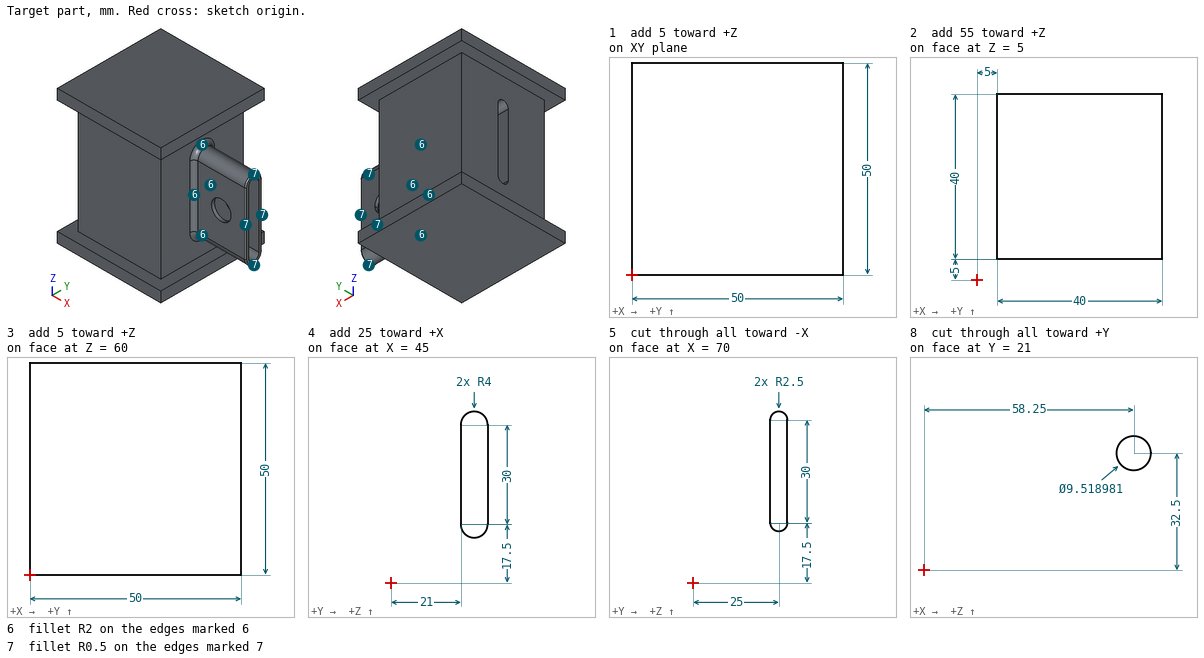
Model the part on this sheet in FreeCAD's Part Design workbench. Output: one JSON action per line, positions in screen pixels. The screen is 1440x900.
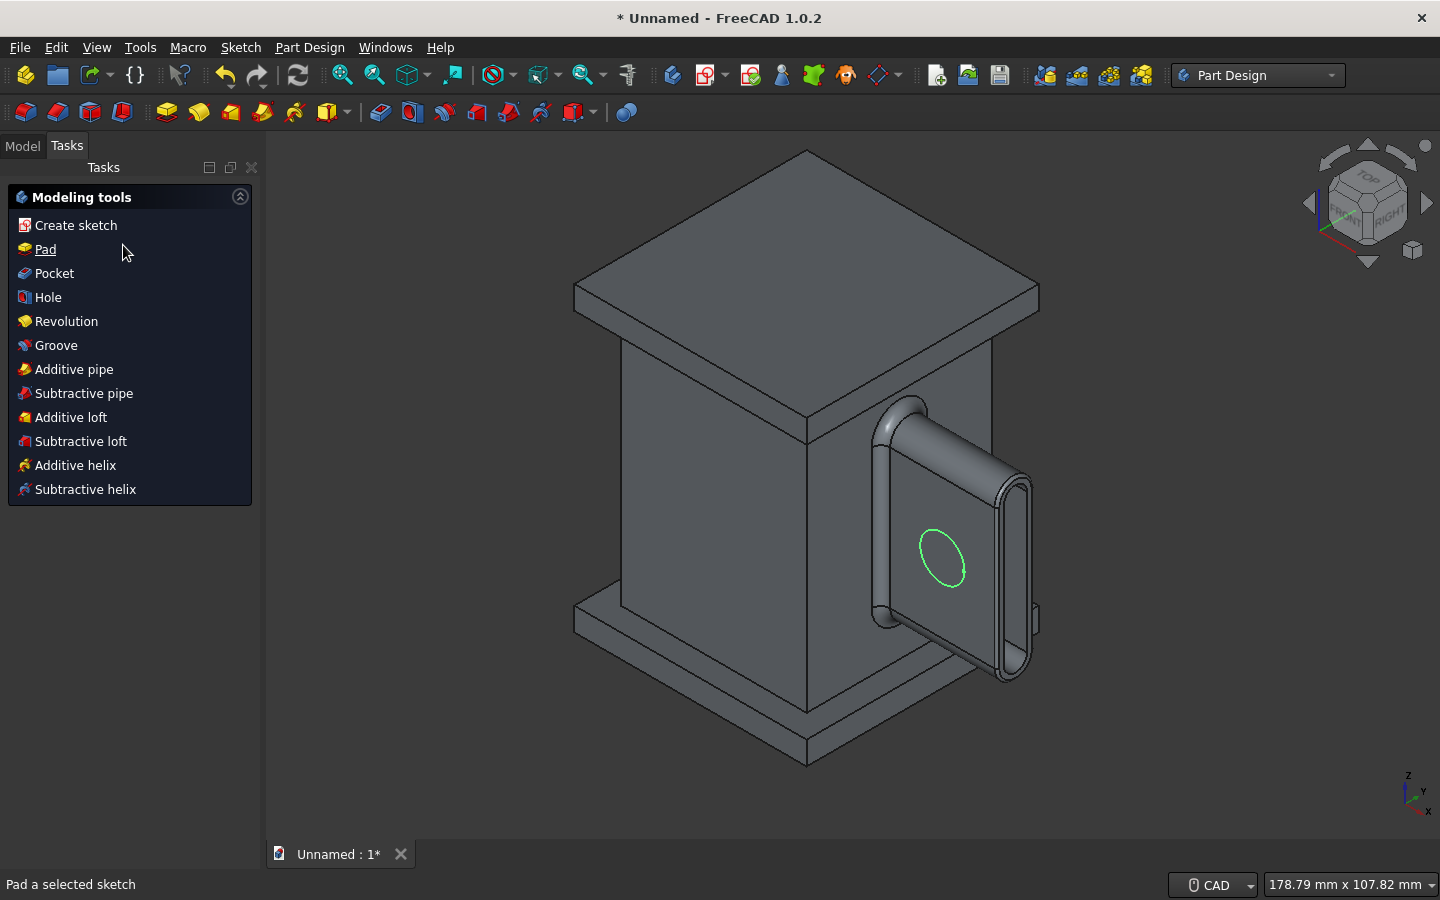
{"action": "left_click", "coordinate": [382, 112]}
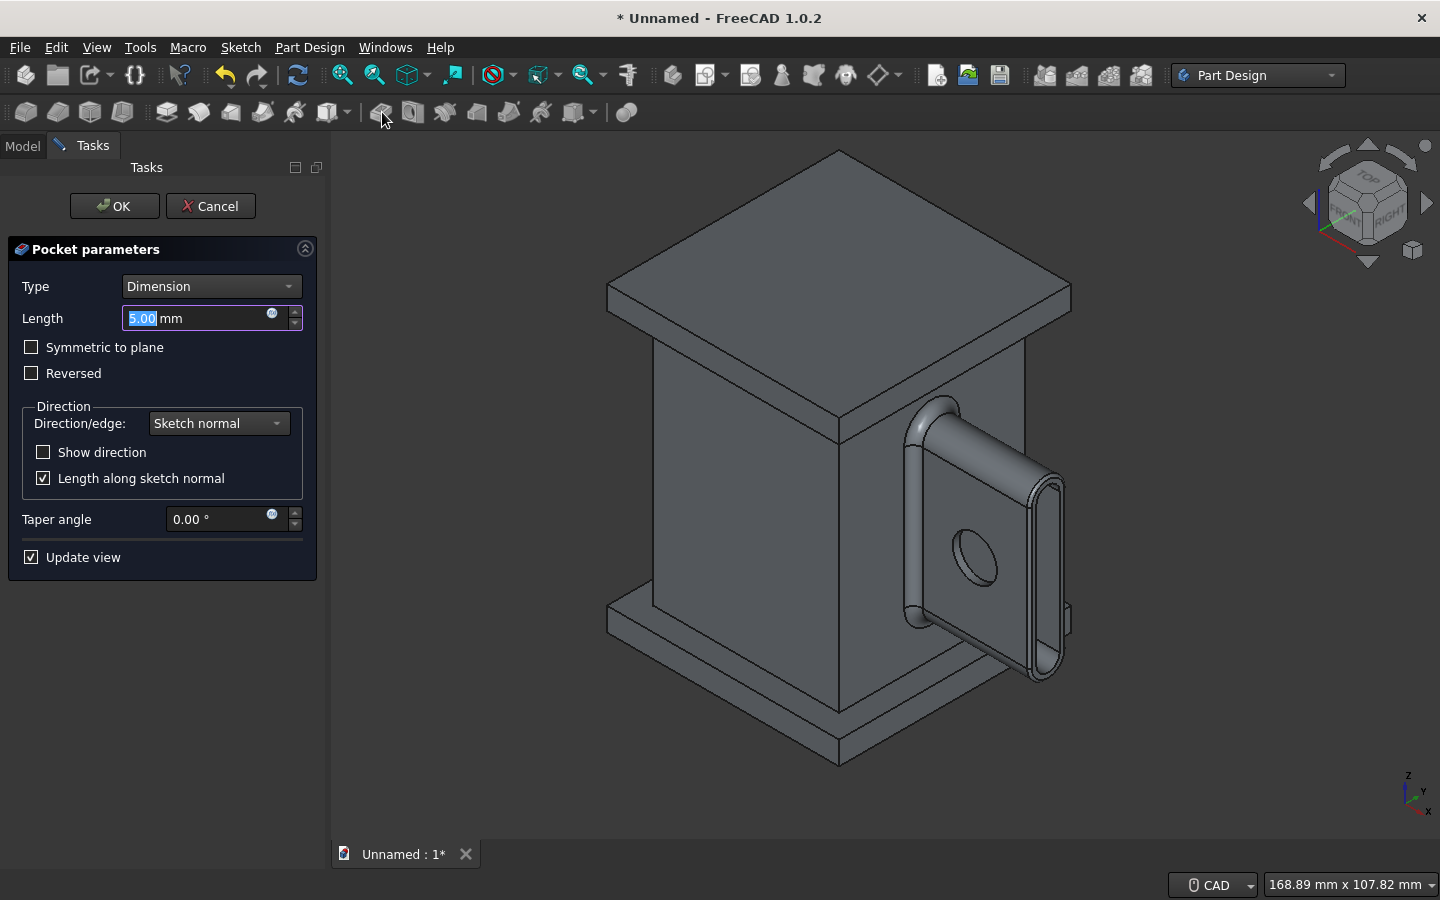
{"action": "left_click", "coordinate": [212, 286]}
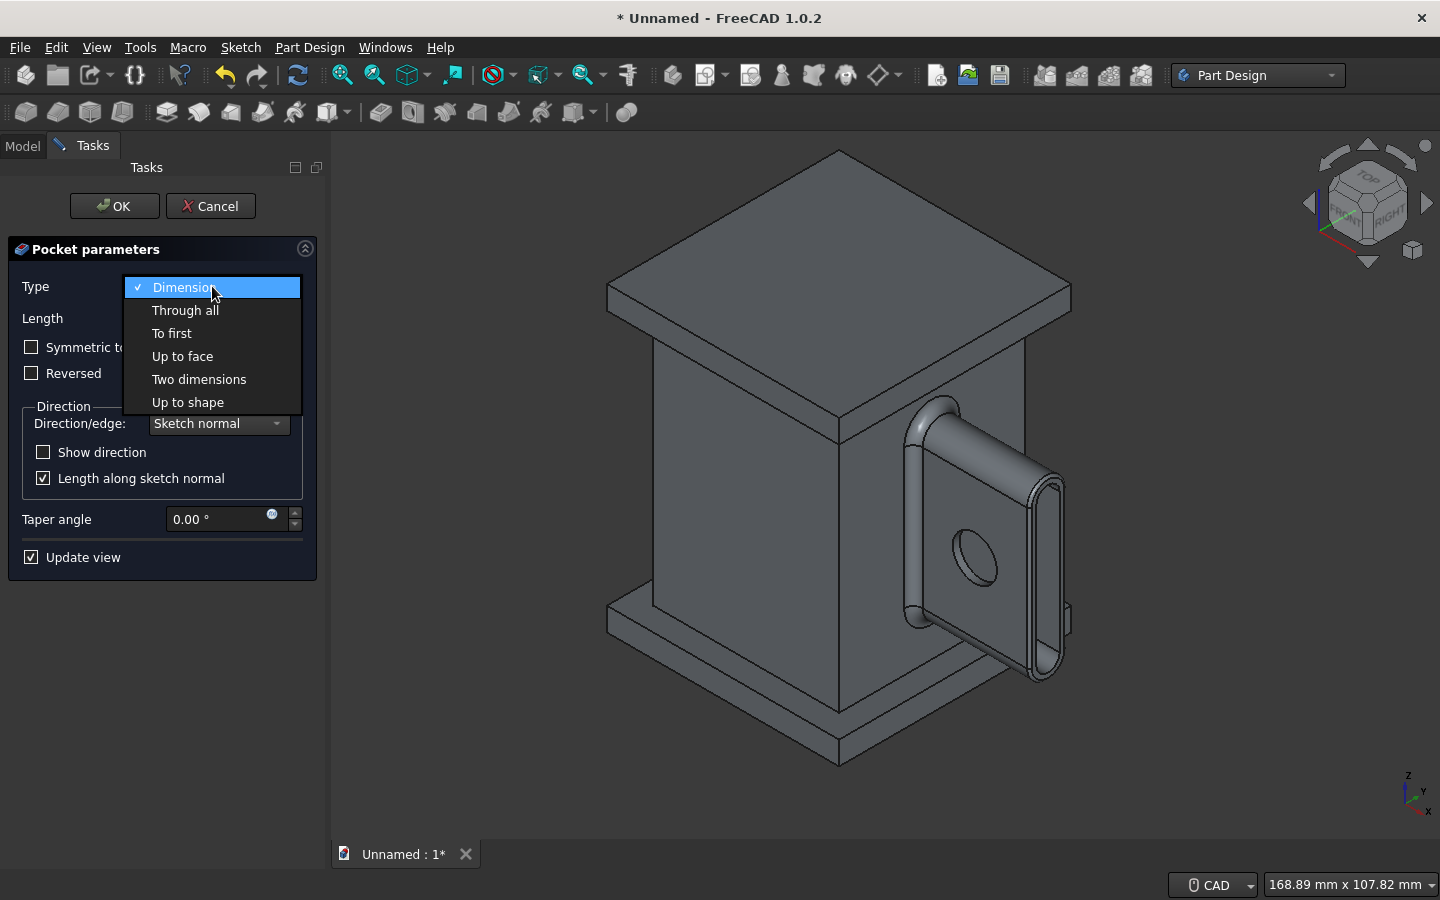
{"action": "left_click", "coordinate": [212, 310]}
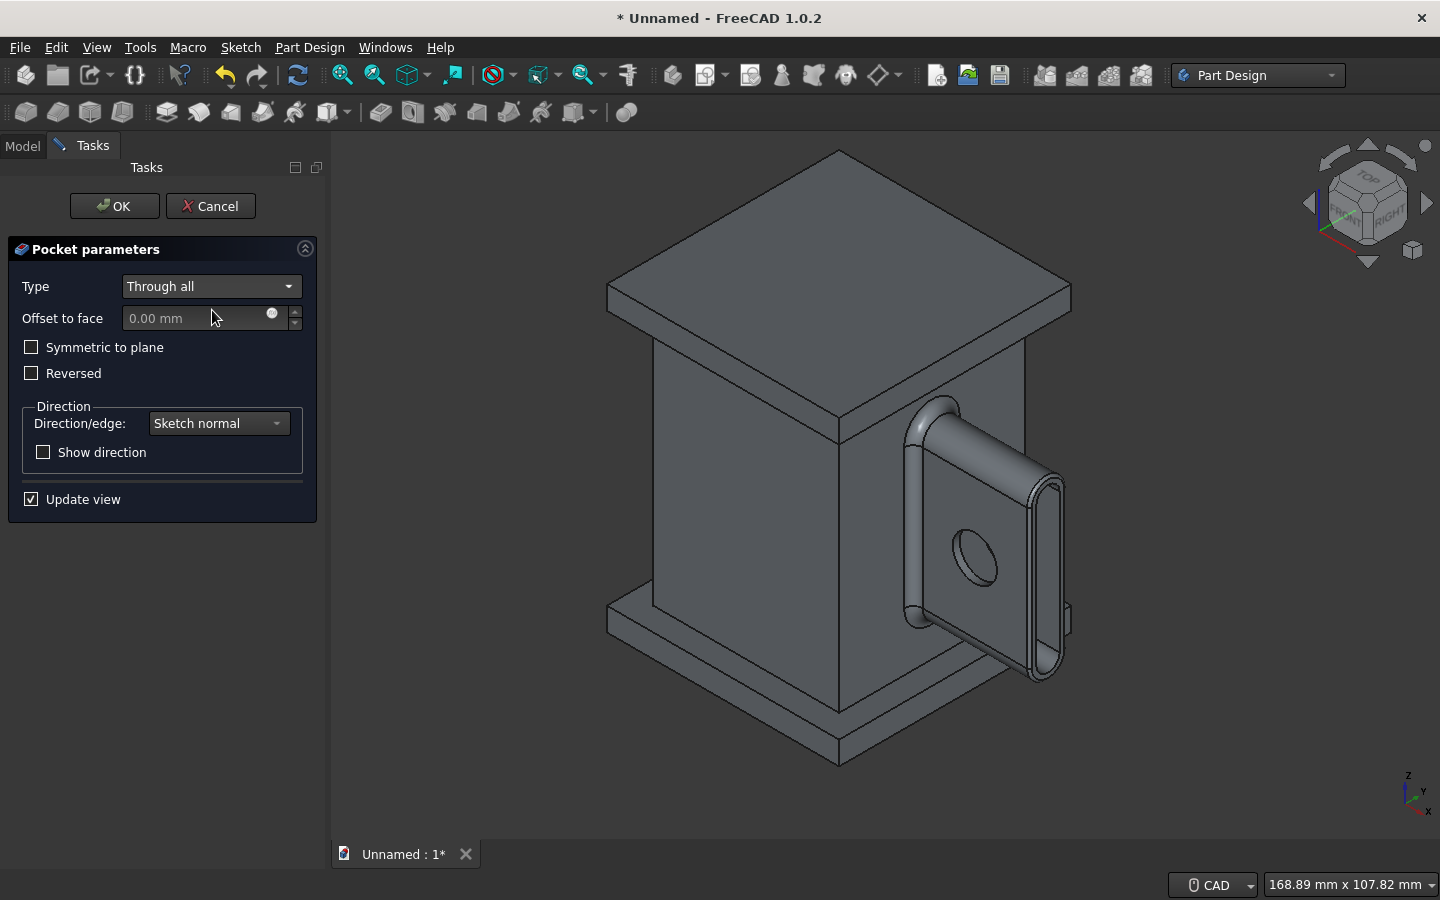
{"action": "left_click", "coordinate": [115, 206]}